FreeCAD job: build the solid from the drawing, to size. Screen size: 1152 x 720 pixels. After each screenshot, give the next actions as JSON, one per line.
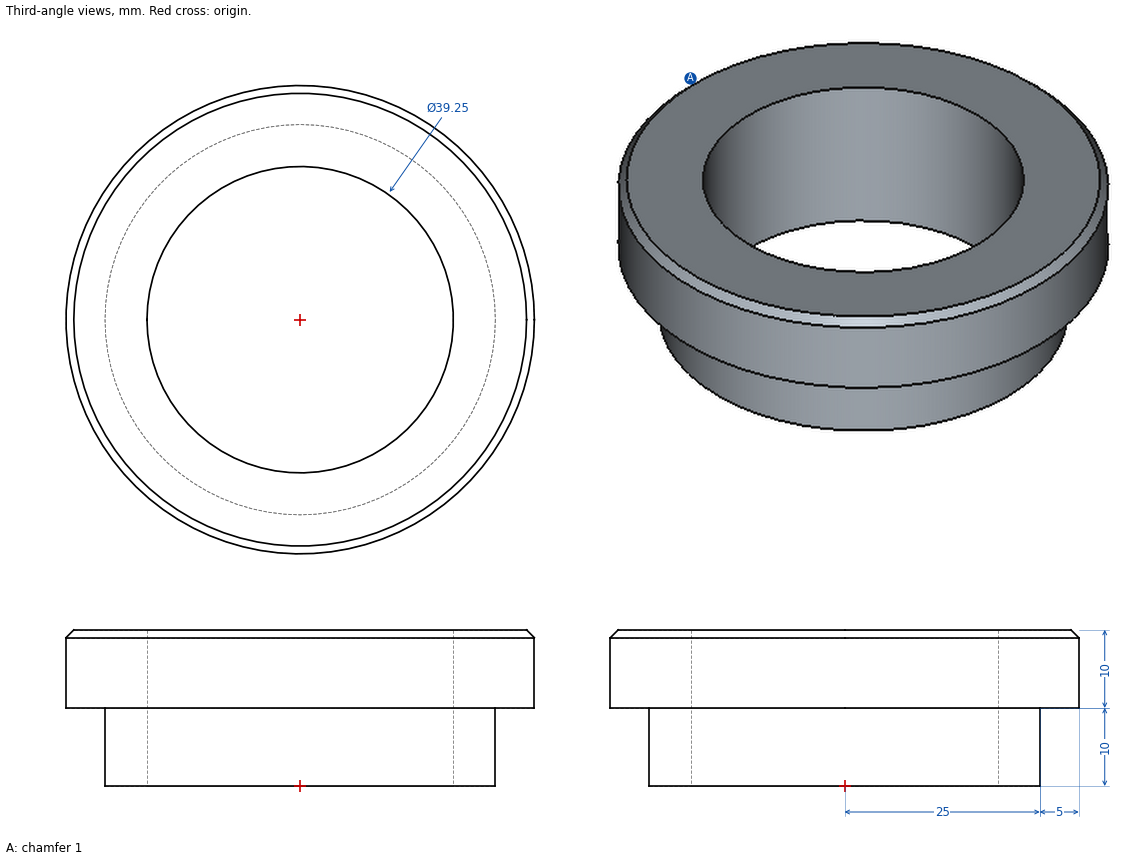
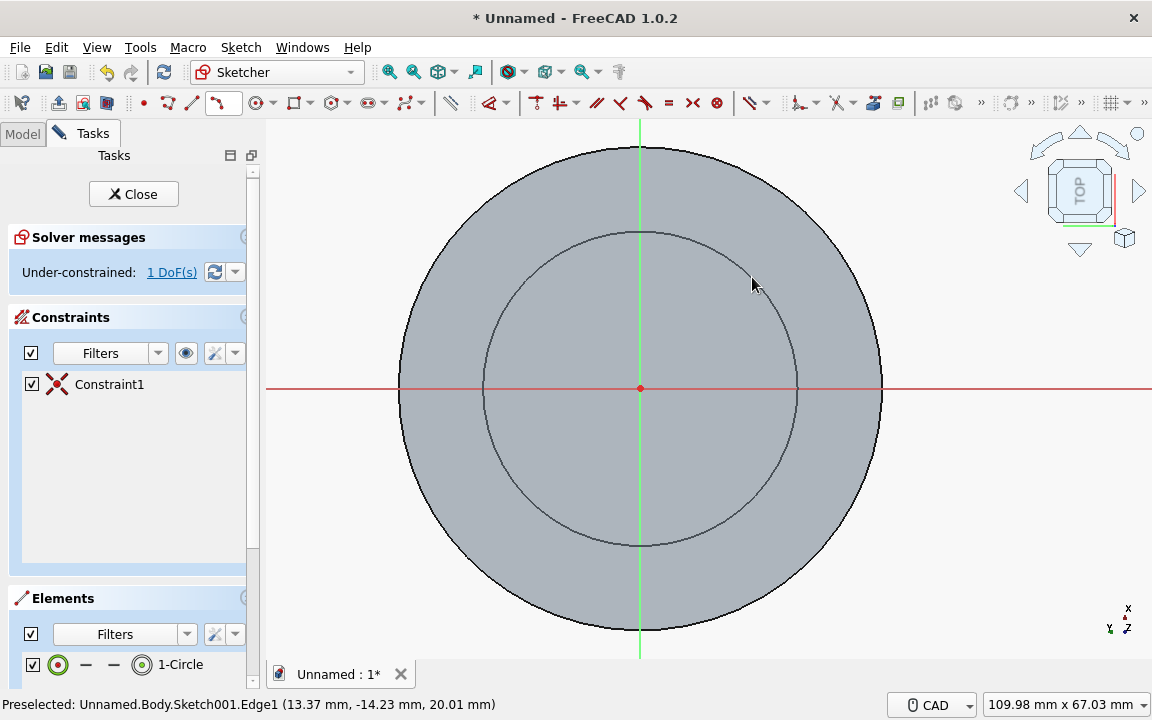
{"action": "key", "text": "d"}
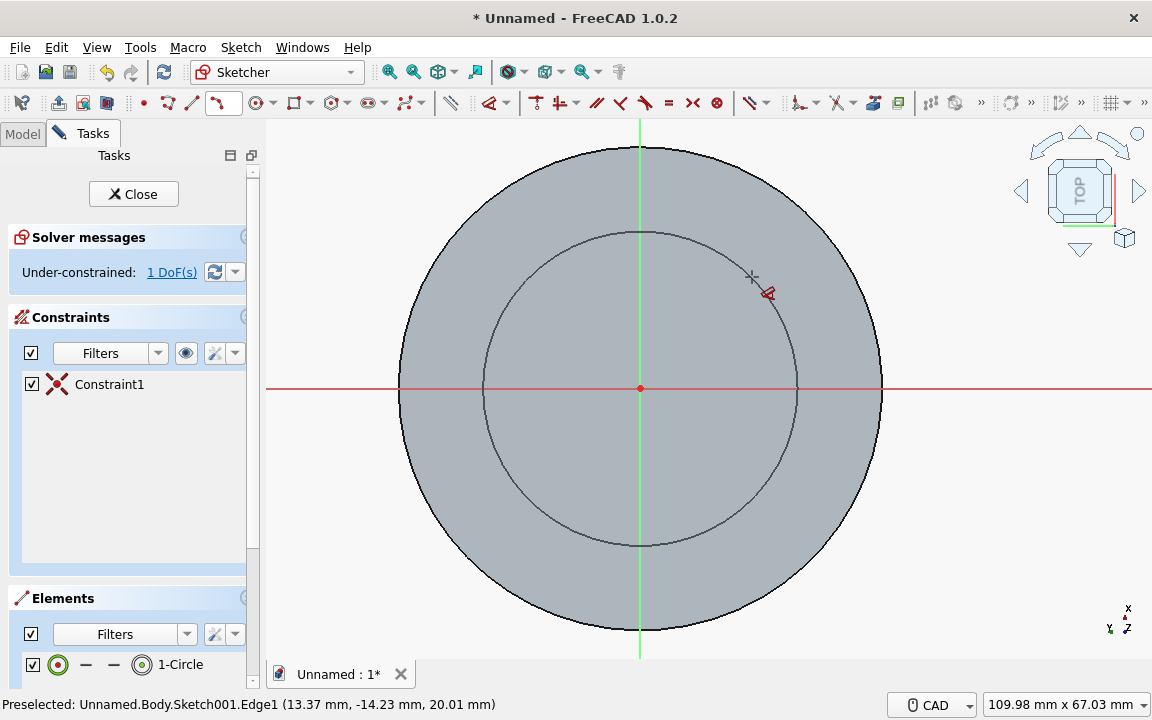
{"action": "left_click", "coordinate": [751, 277]}
{"action": "left_click", "coordinate": [774, 254]}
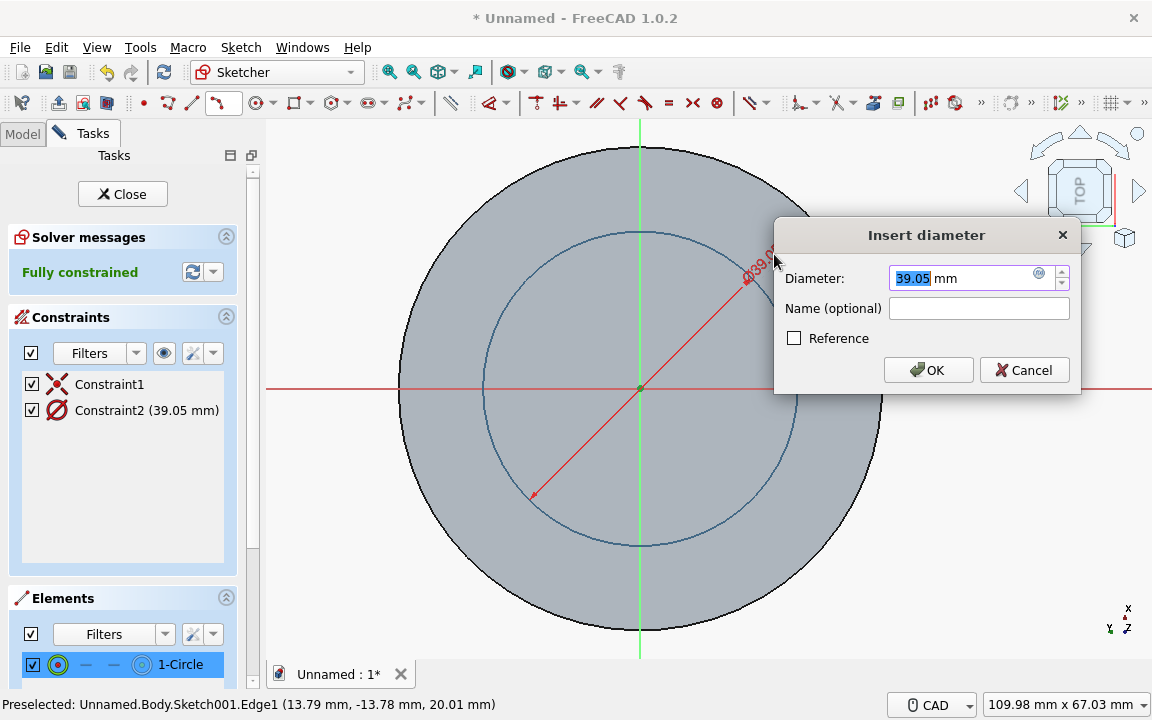
{"action": "type", "text": "39.25"}
{"action": "key", "text": "Return"}
{"action": "key", "text": "Escape"}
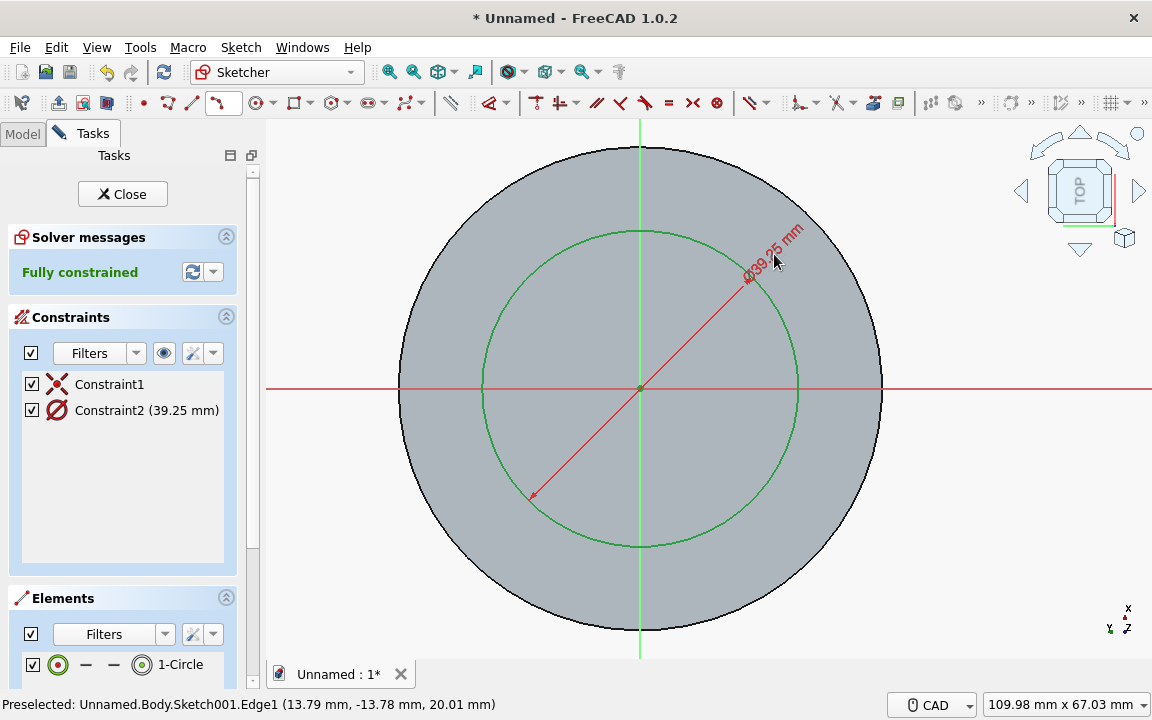
{"action": "left_click", "coordinate": [123, 194]}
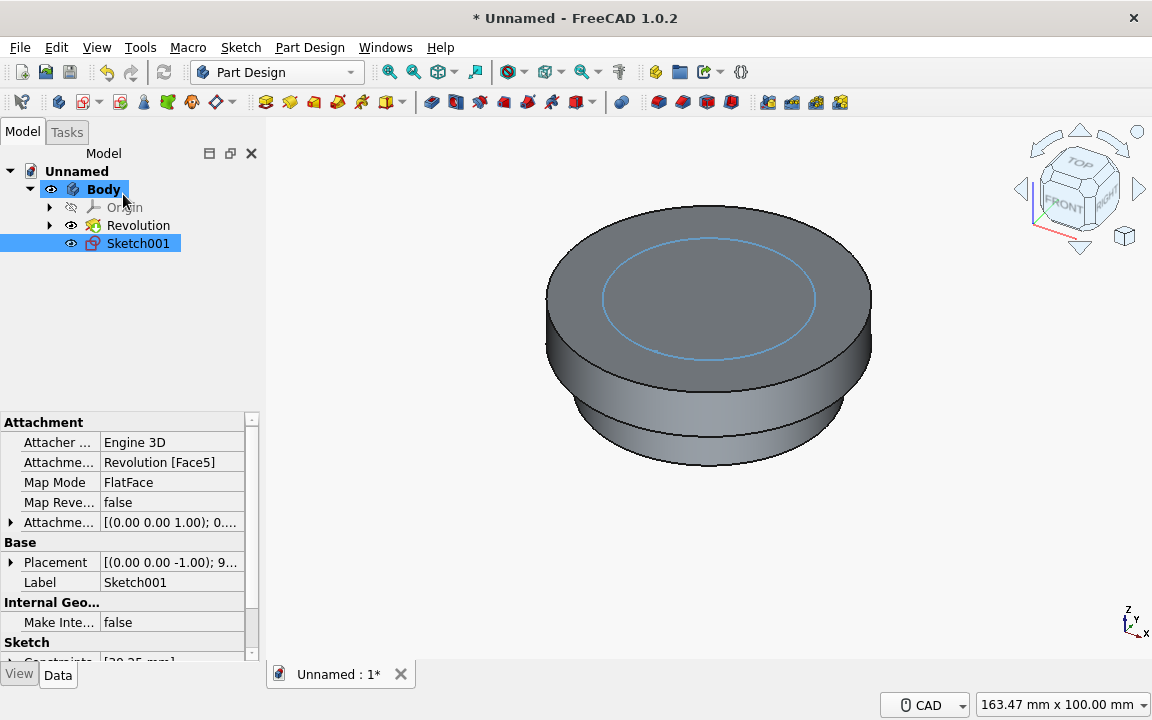
{"action": "left_click", "coordinate": [432, 102]}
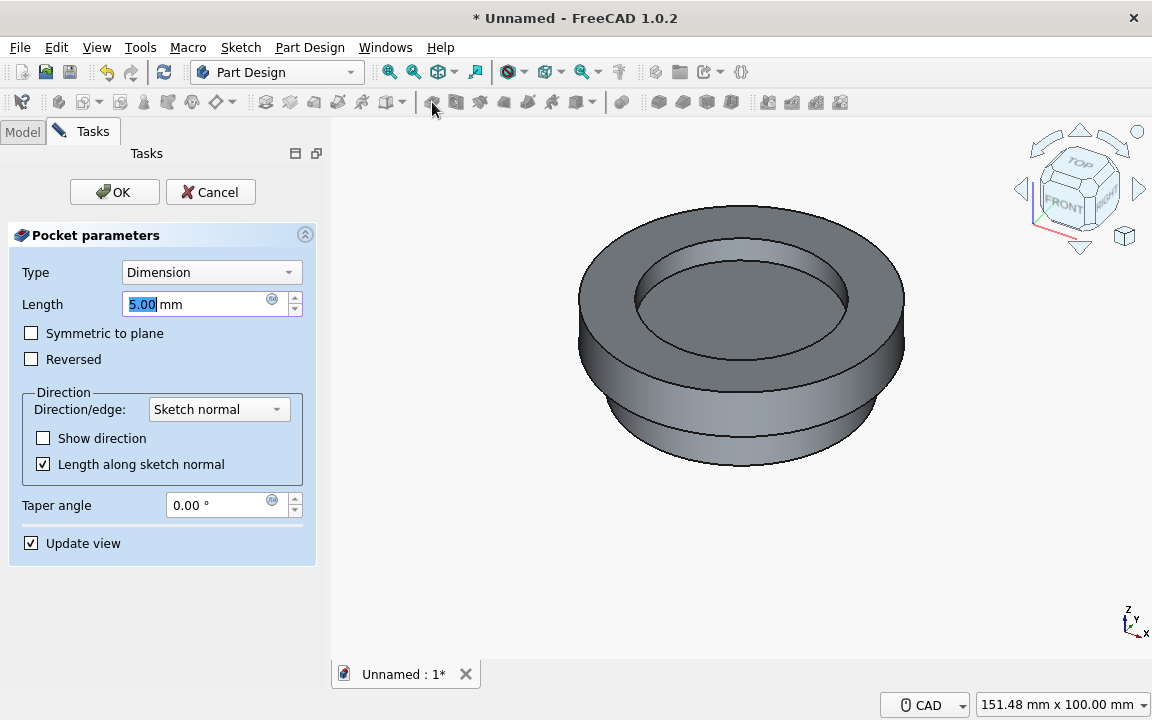
{"action": "left_click", "coordinate": [212, 272]}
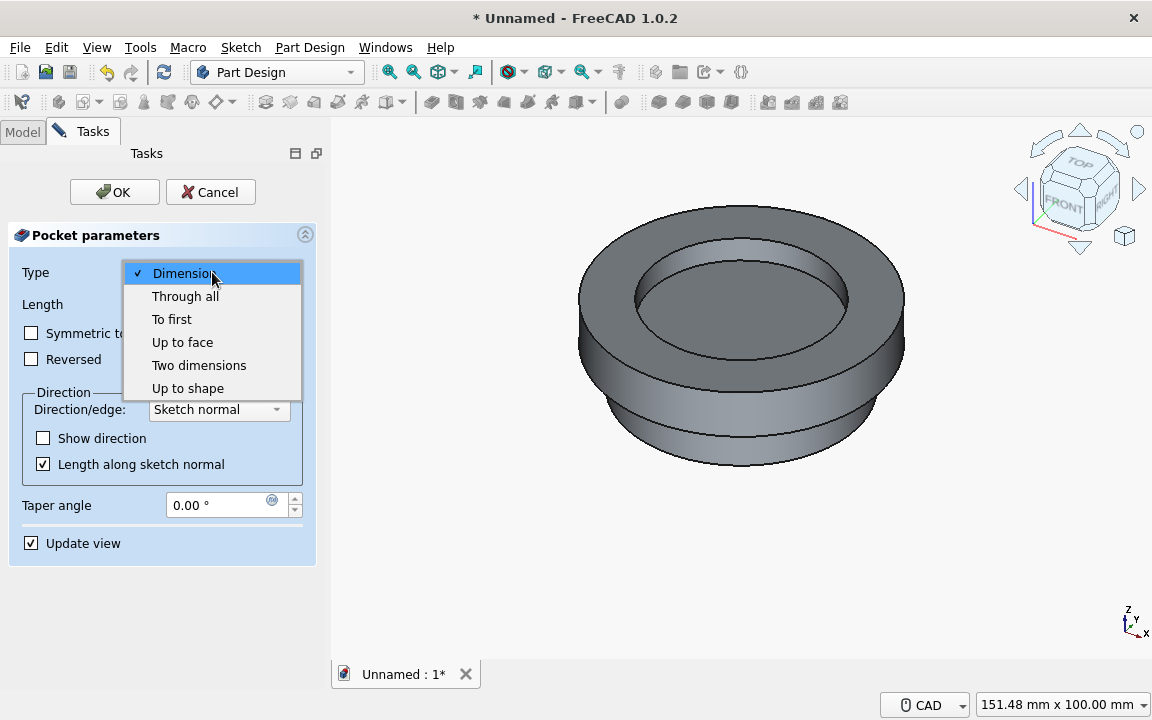
{"action": "left_click", "coordinate": [212, 296]}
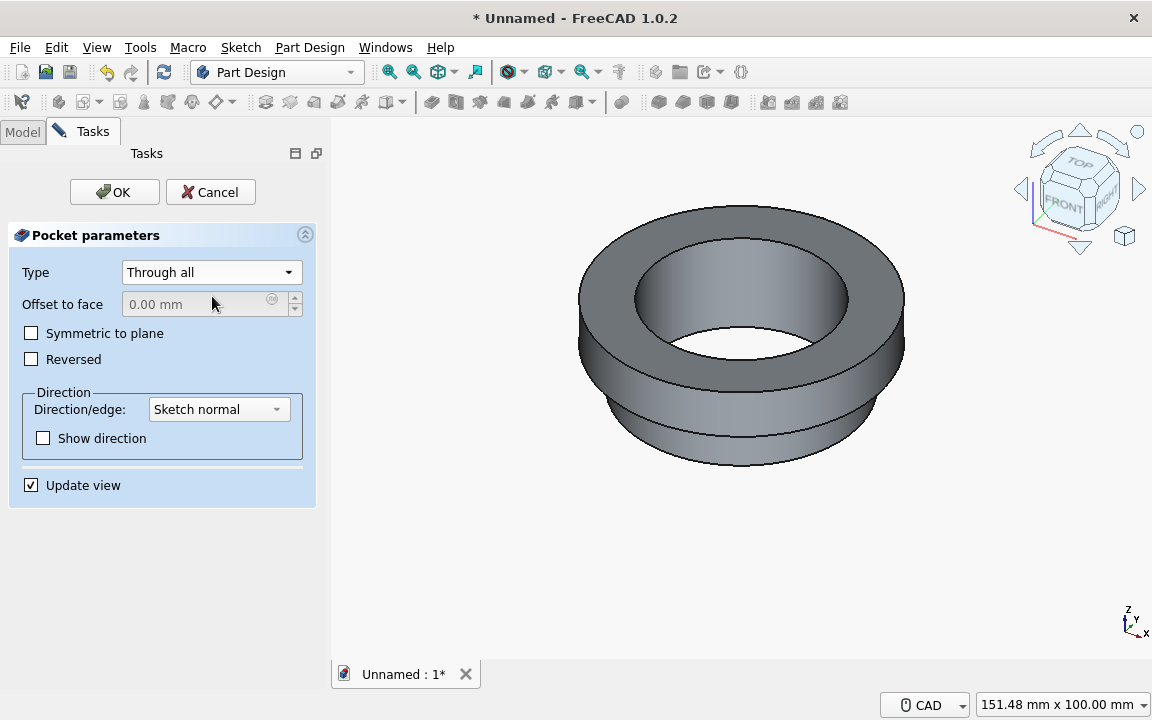
{"action": "left_click", "coordinate": [115, 192]}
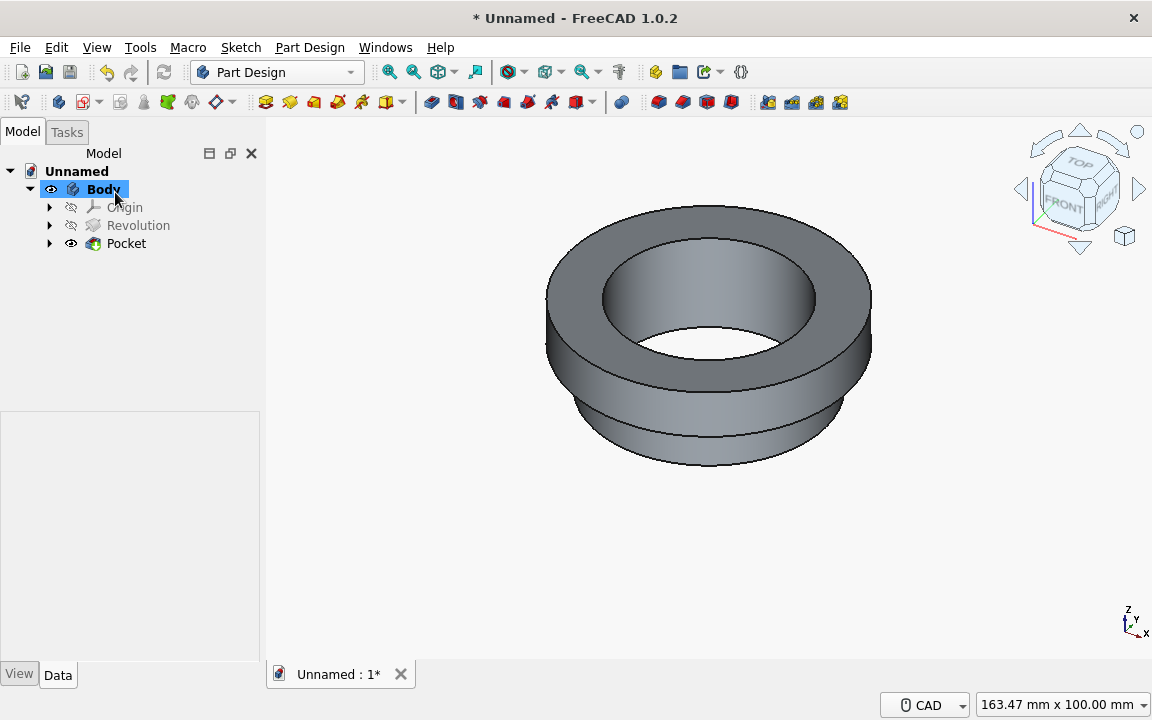
{"action": "left_click", "coordinate": [628, 379]}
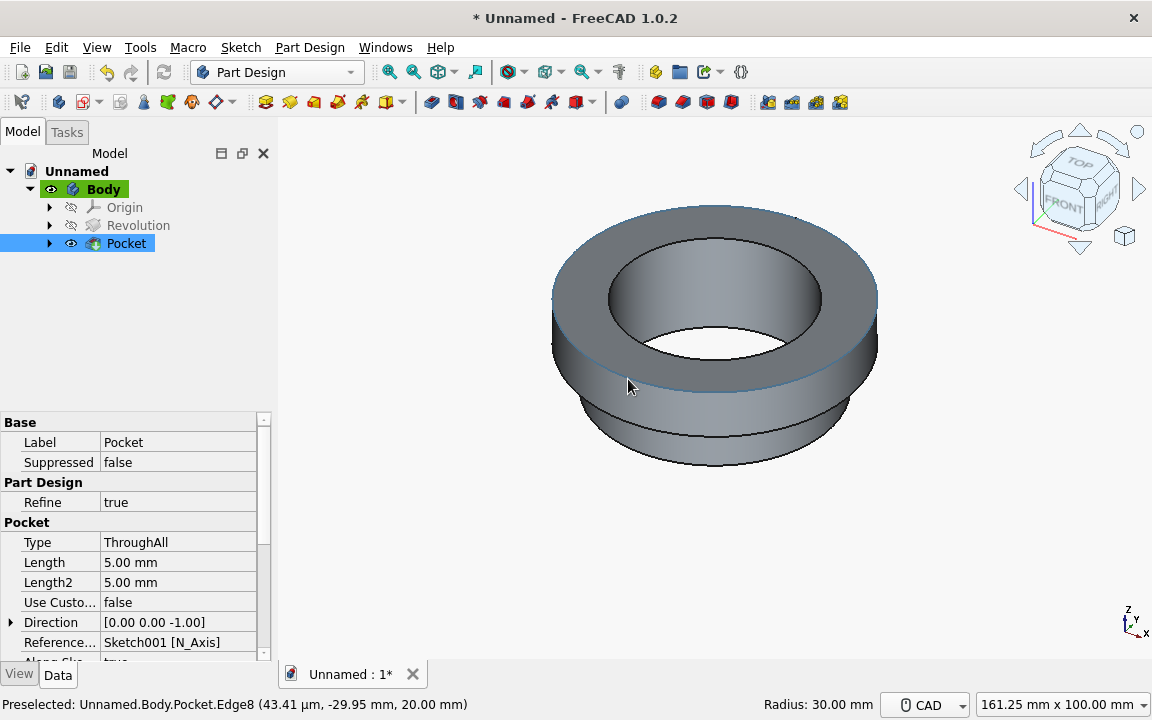
{"action": "left_click", "coordinate": [684, 102]}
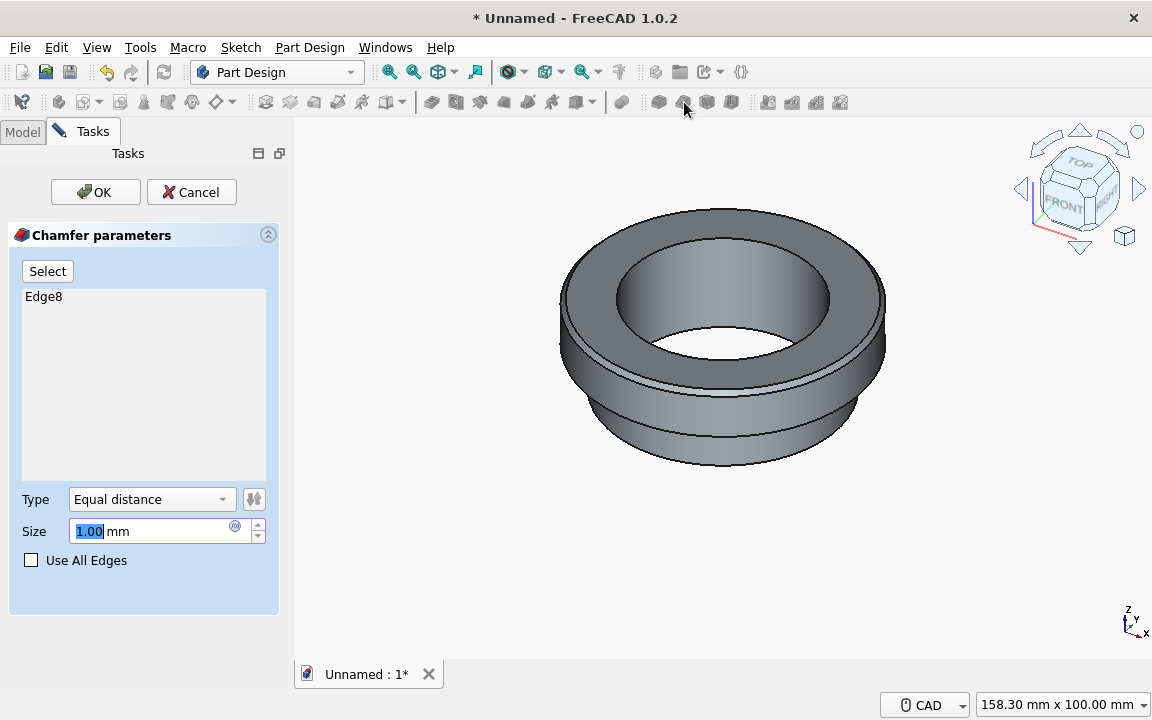
{"action": "type", "text": "1"}
{"action": "key", "text": "Tab"}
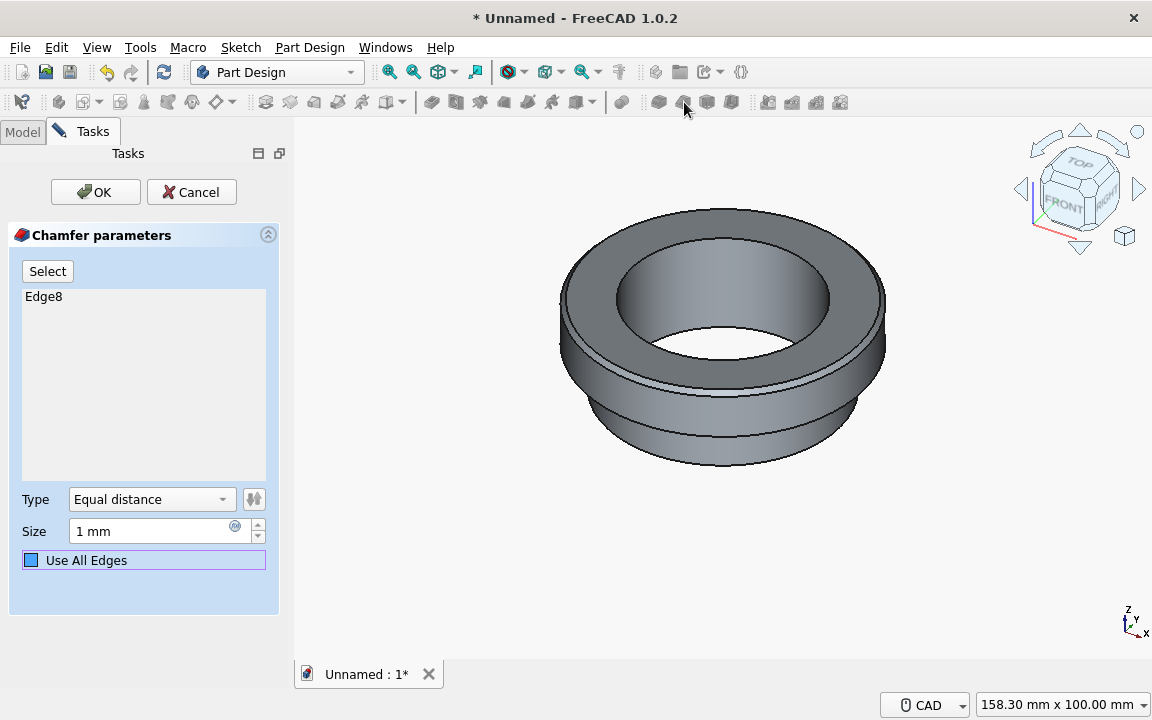
{"action": "left_click", "coordinate": [96, 192]}